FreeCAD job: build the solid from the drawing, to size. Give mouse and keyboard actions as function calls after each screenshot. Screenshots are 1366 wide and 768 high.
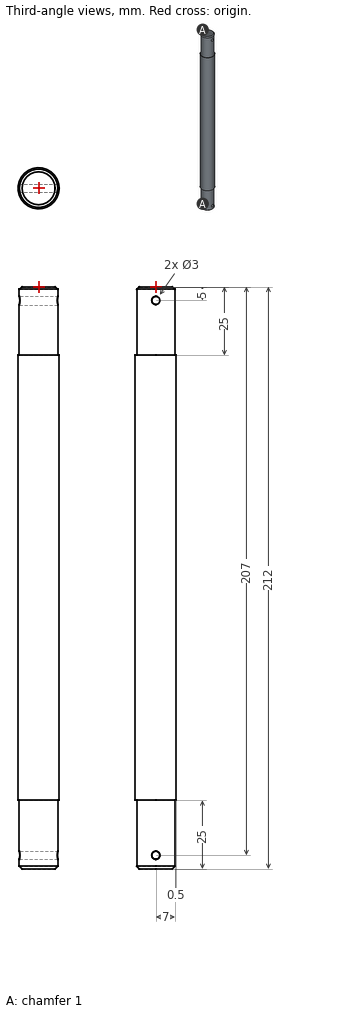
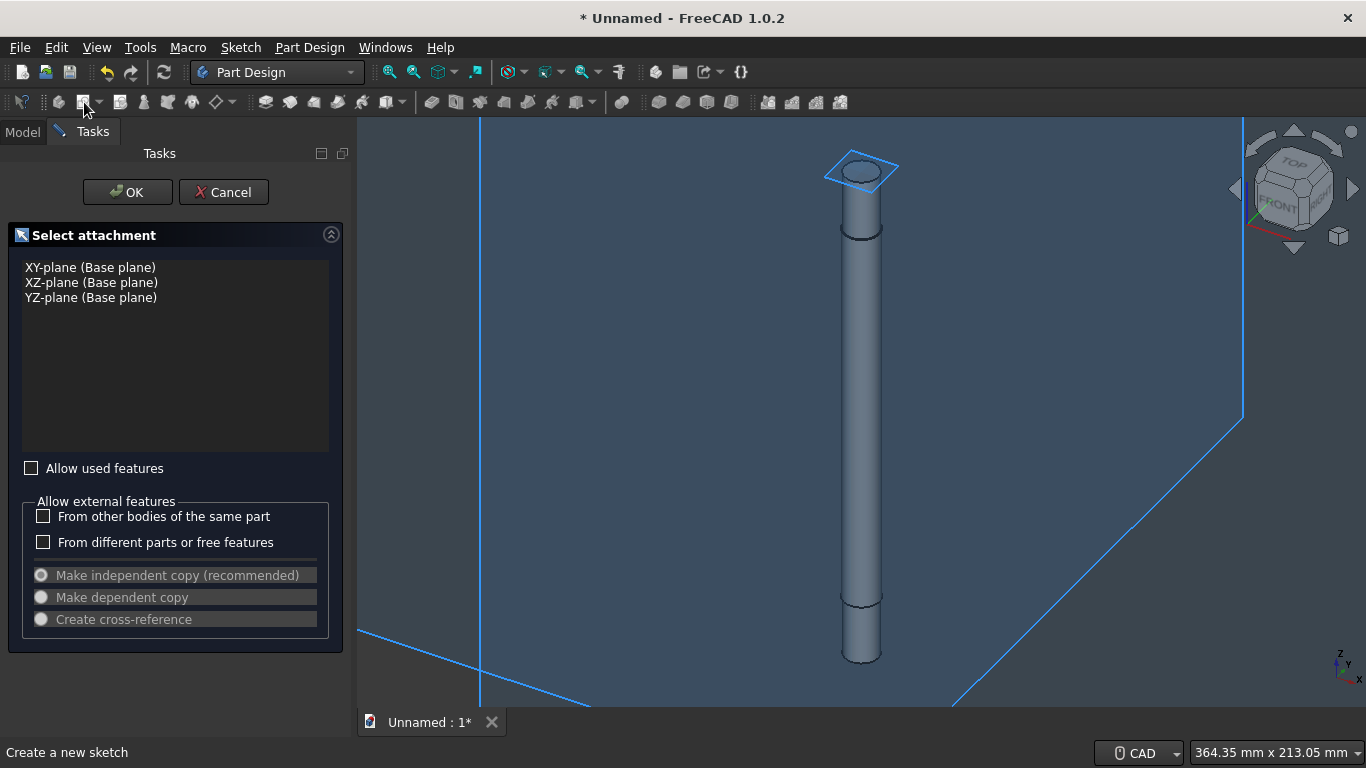
click(82, 298)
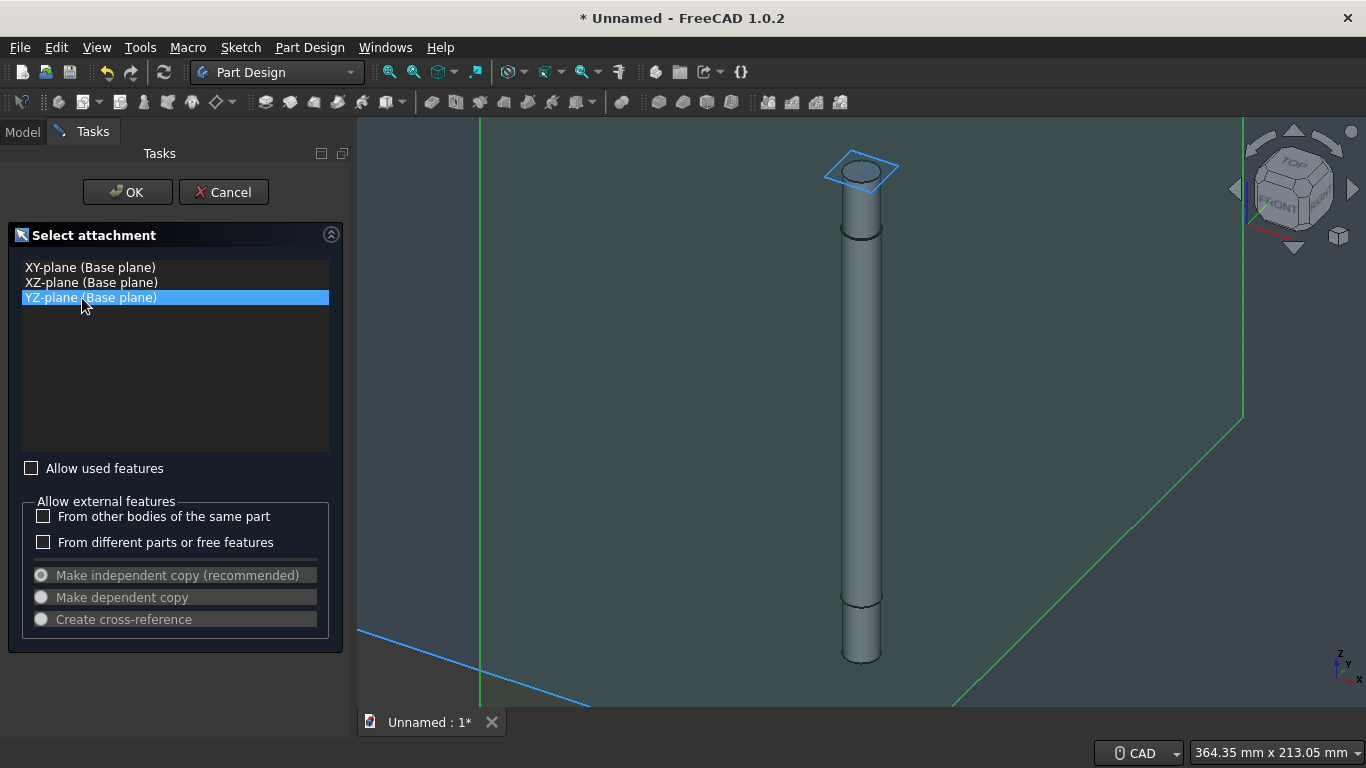
click(128, 192)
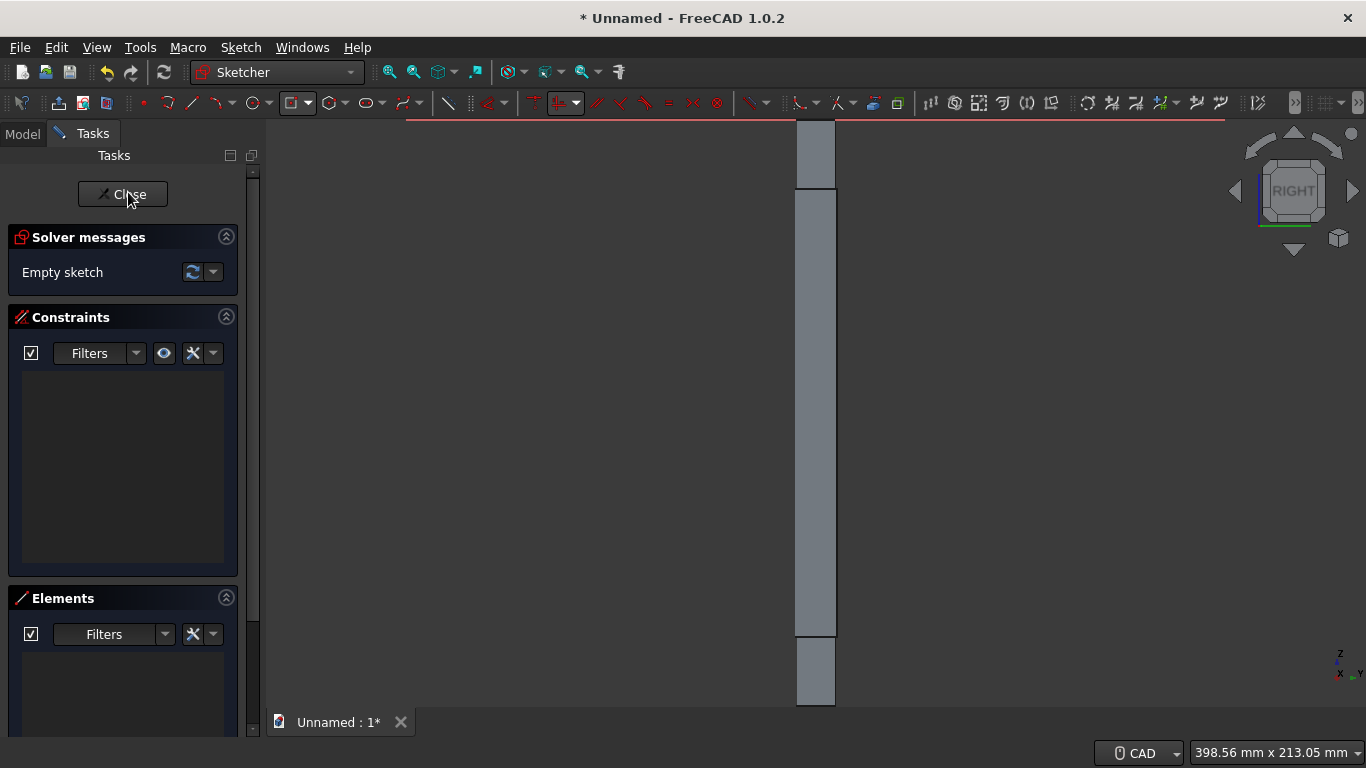
key(q)
key(s)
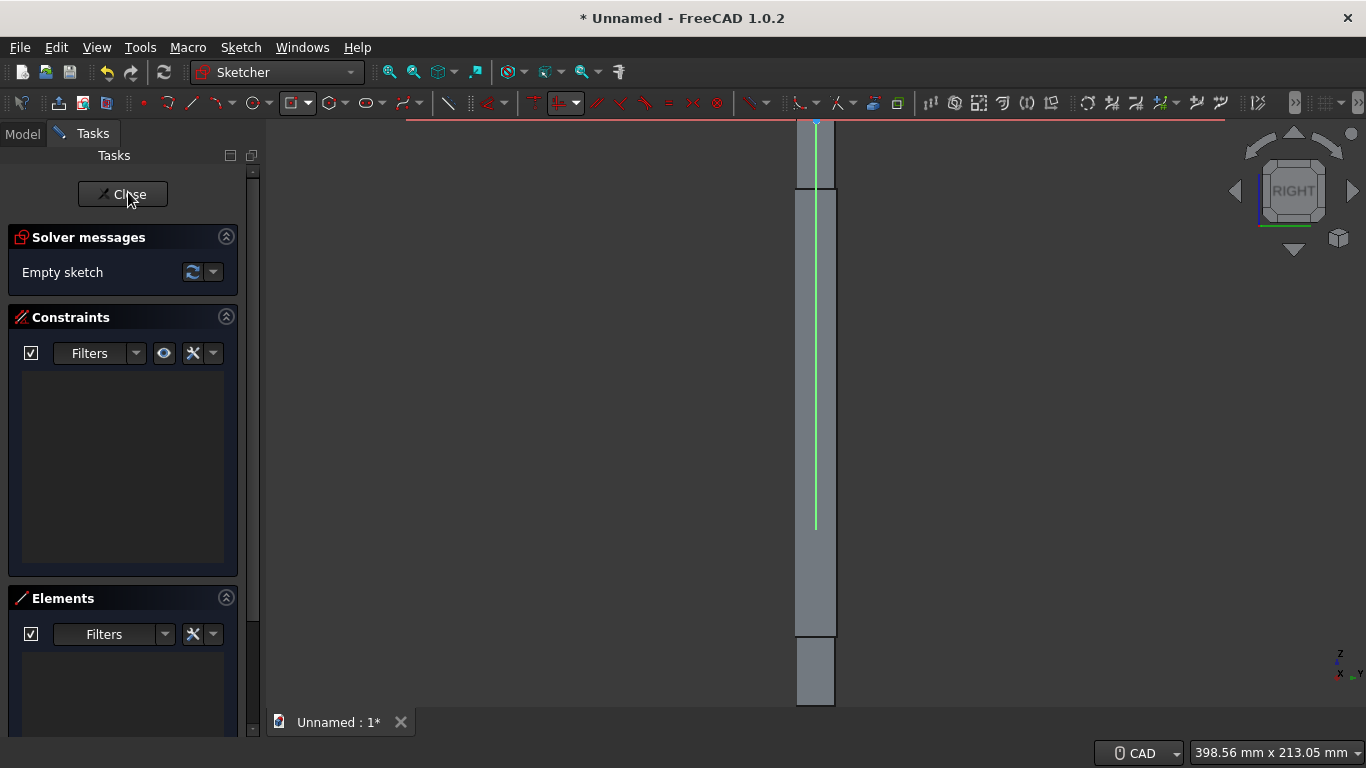
scroll(608, 423, down, 2)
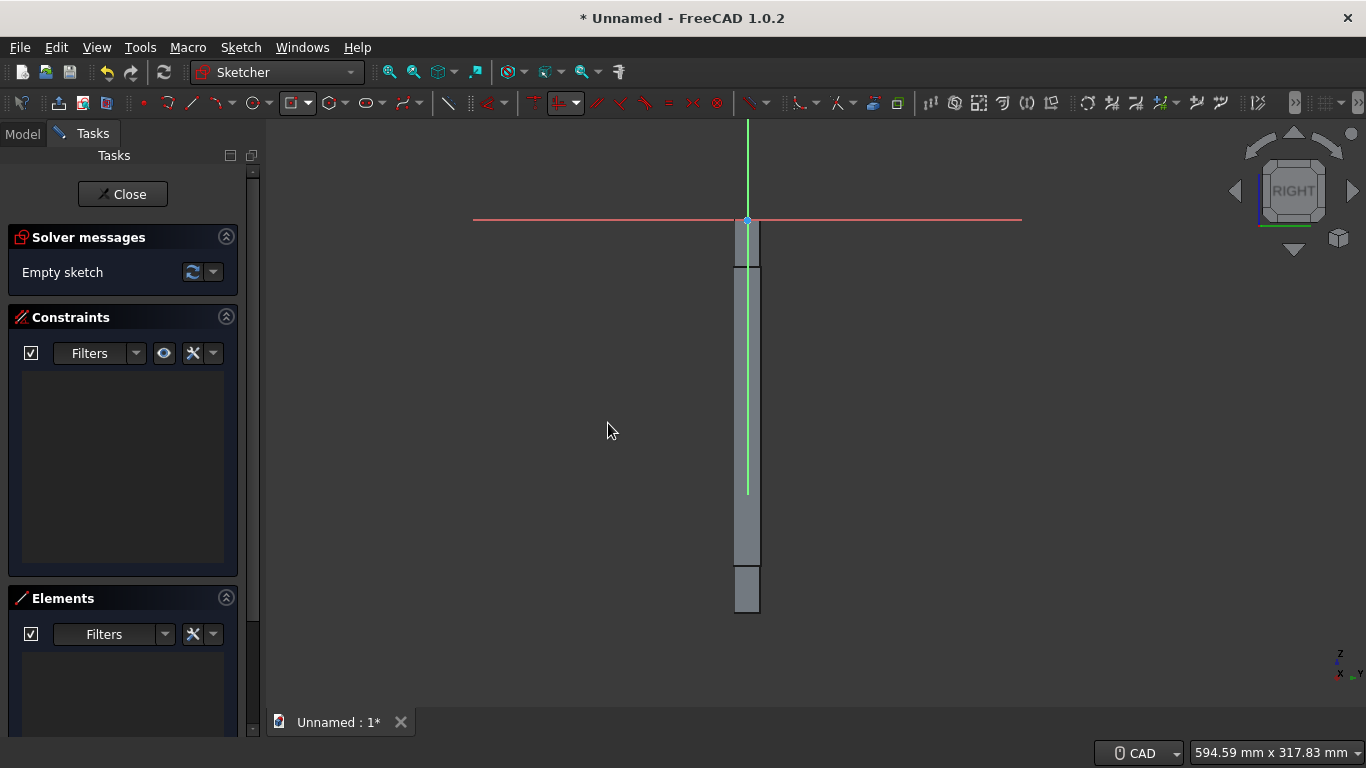
key(g)
key(c)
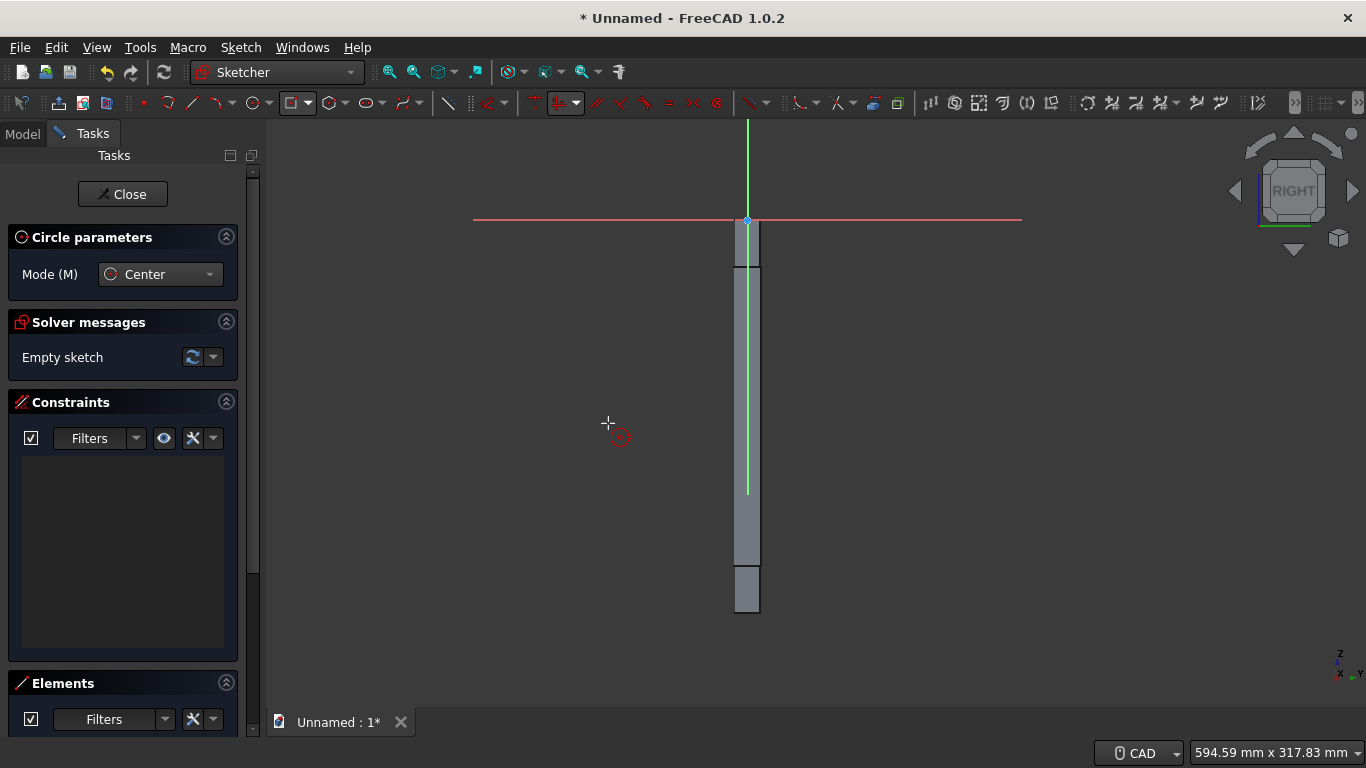
scroll(748, 230, up, 11)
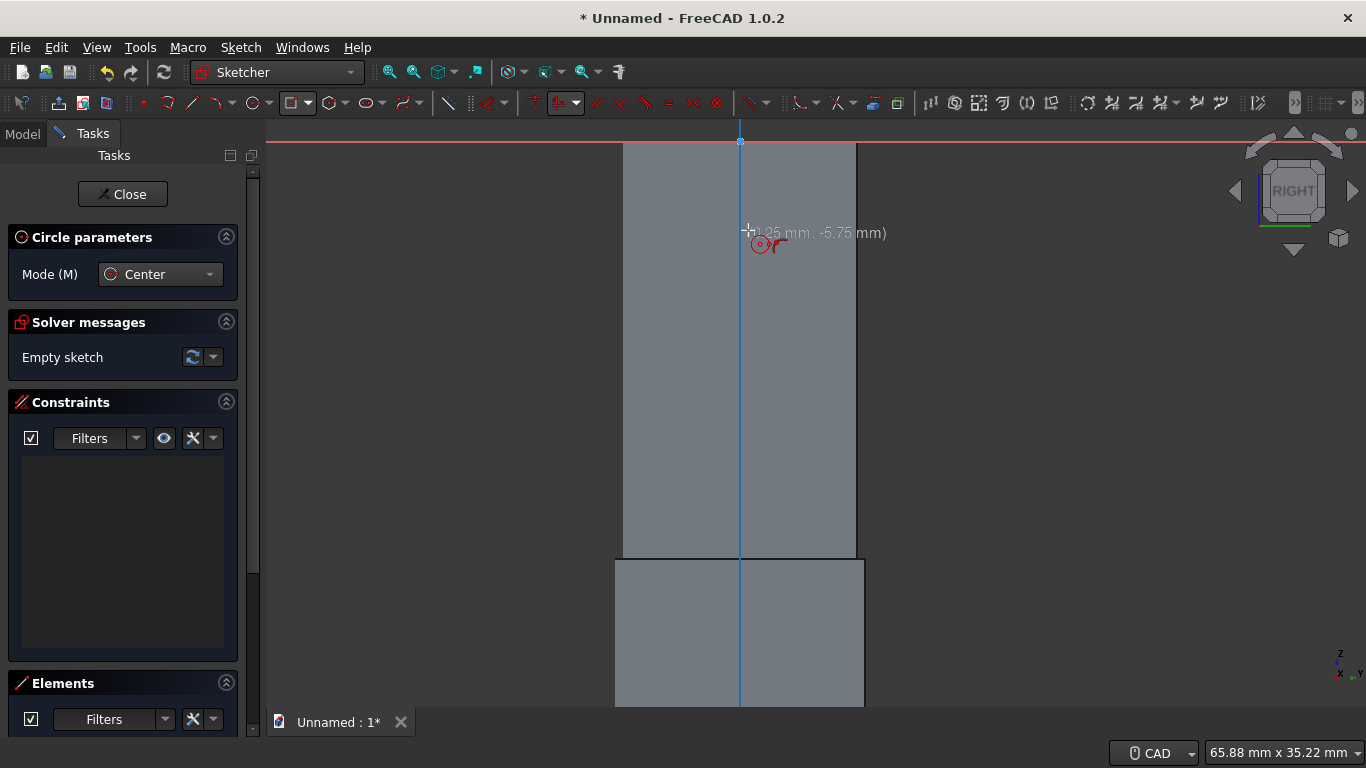
scroll(748, 230, down, 11)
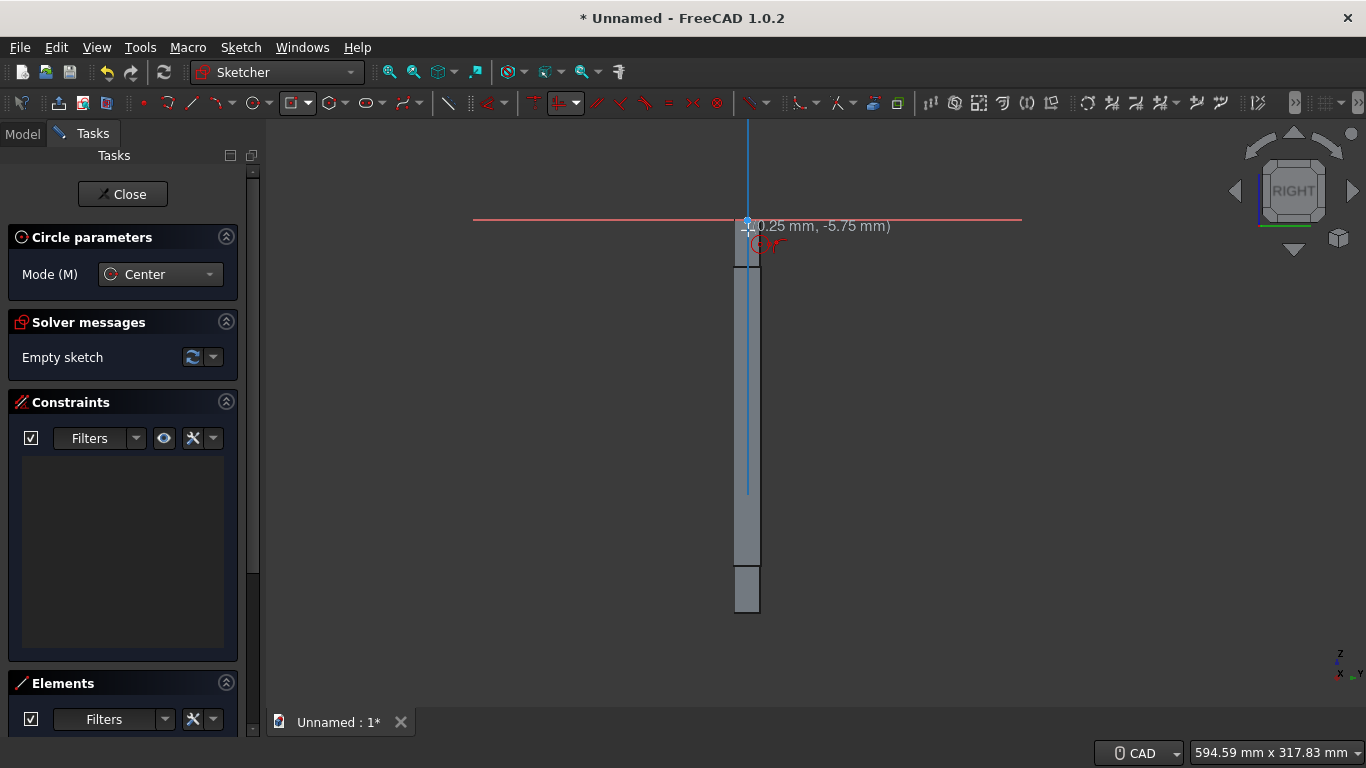
scroll(748, 230, up, 3)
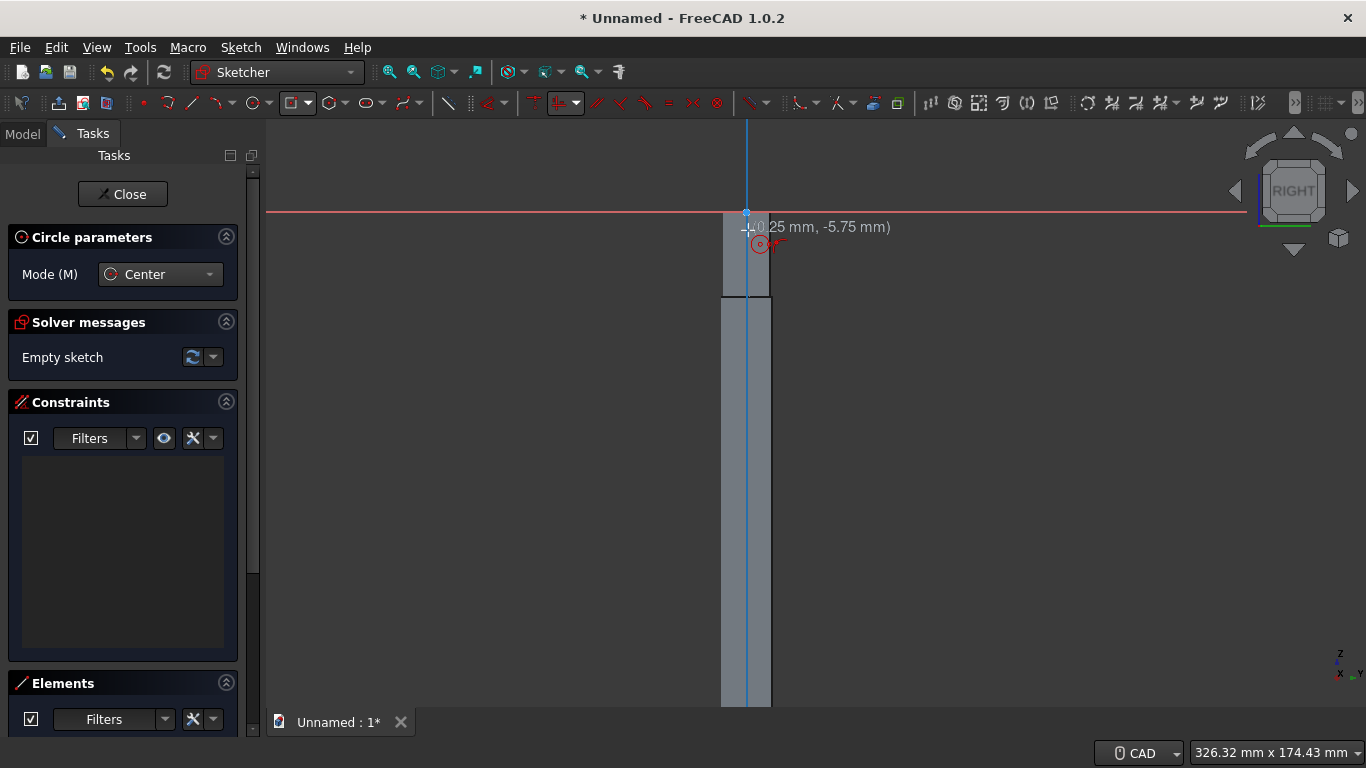
click(747, 229)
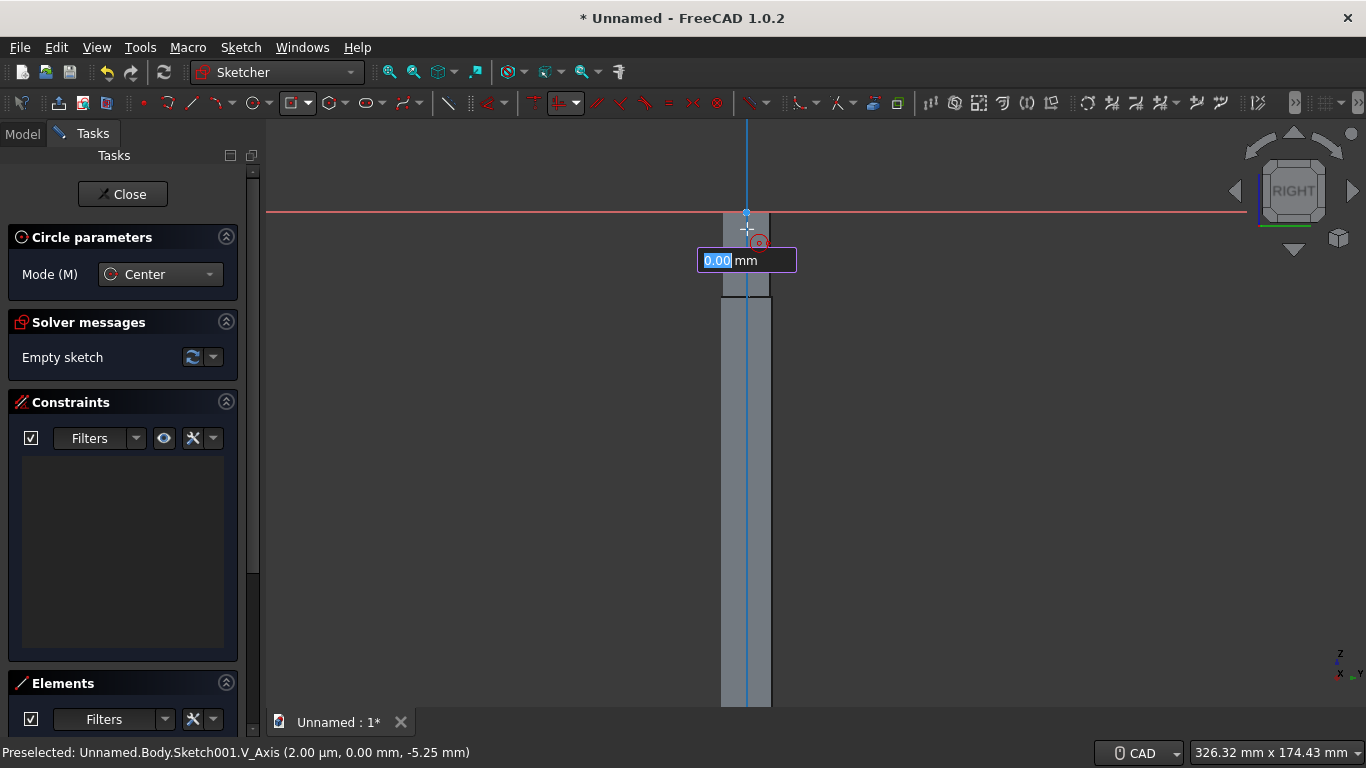
scroll(752, 227, up, 7)
move(749, 228)